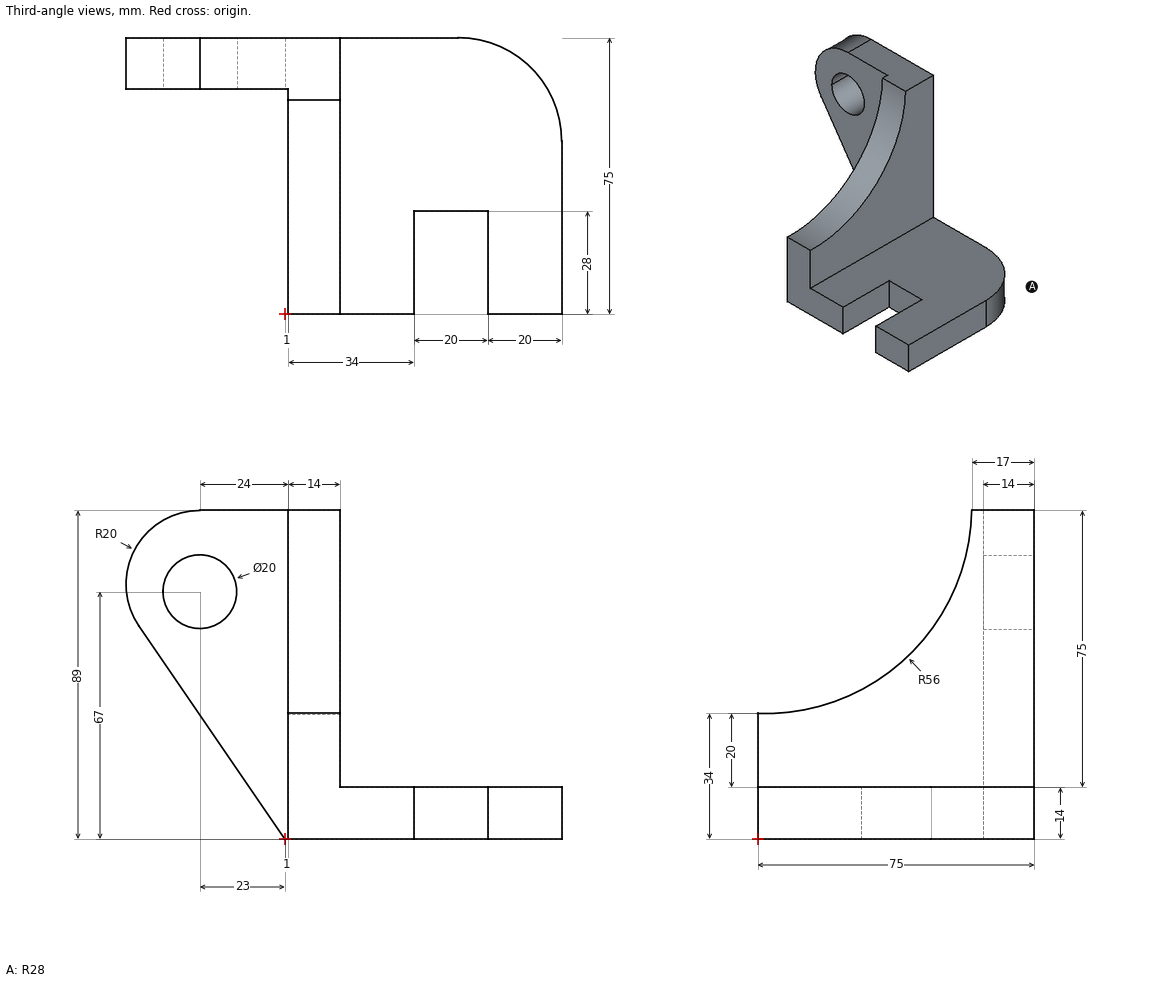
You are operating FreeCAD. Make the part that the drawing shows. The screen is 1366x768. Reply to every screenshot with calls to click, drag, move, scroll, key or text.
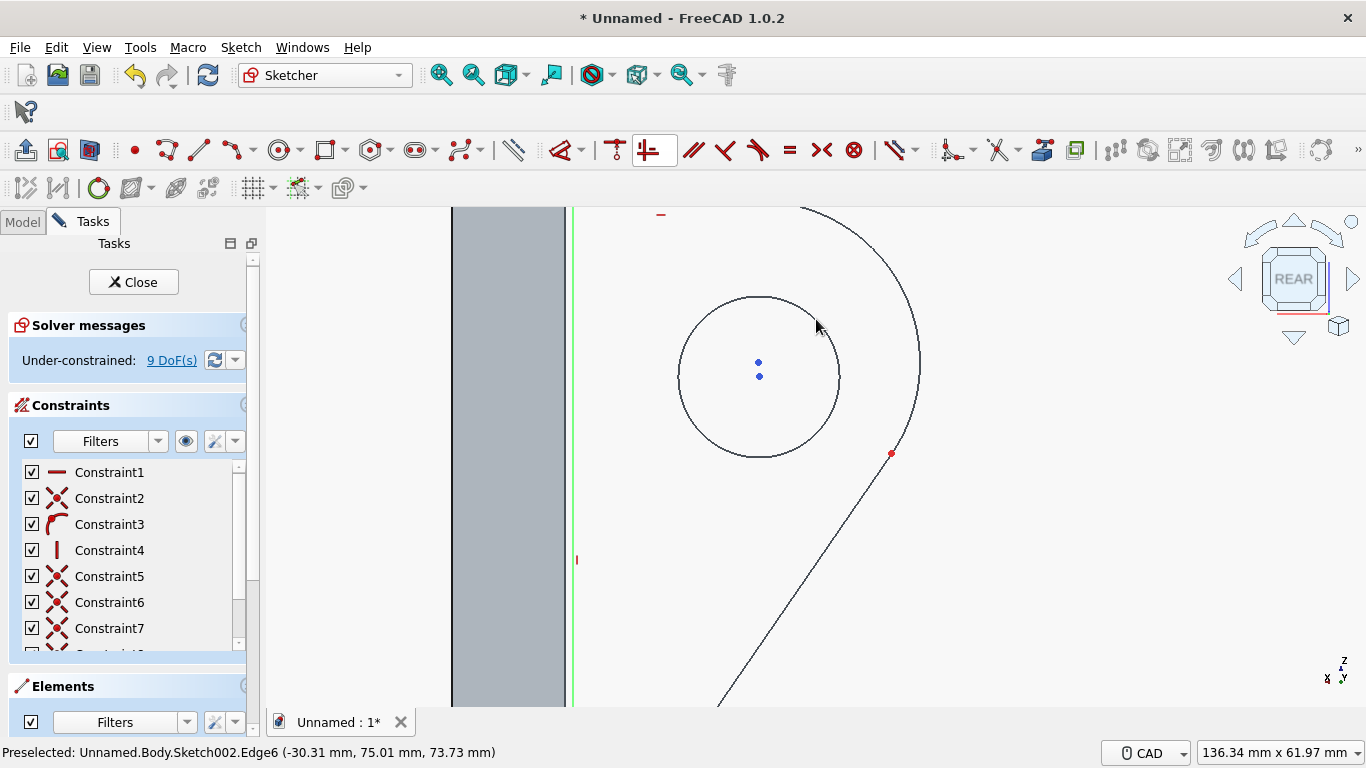
scroll(759, 375, down, 4)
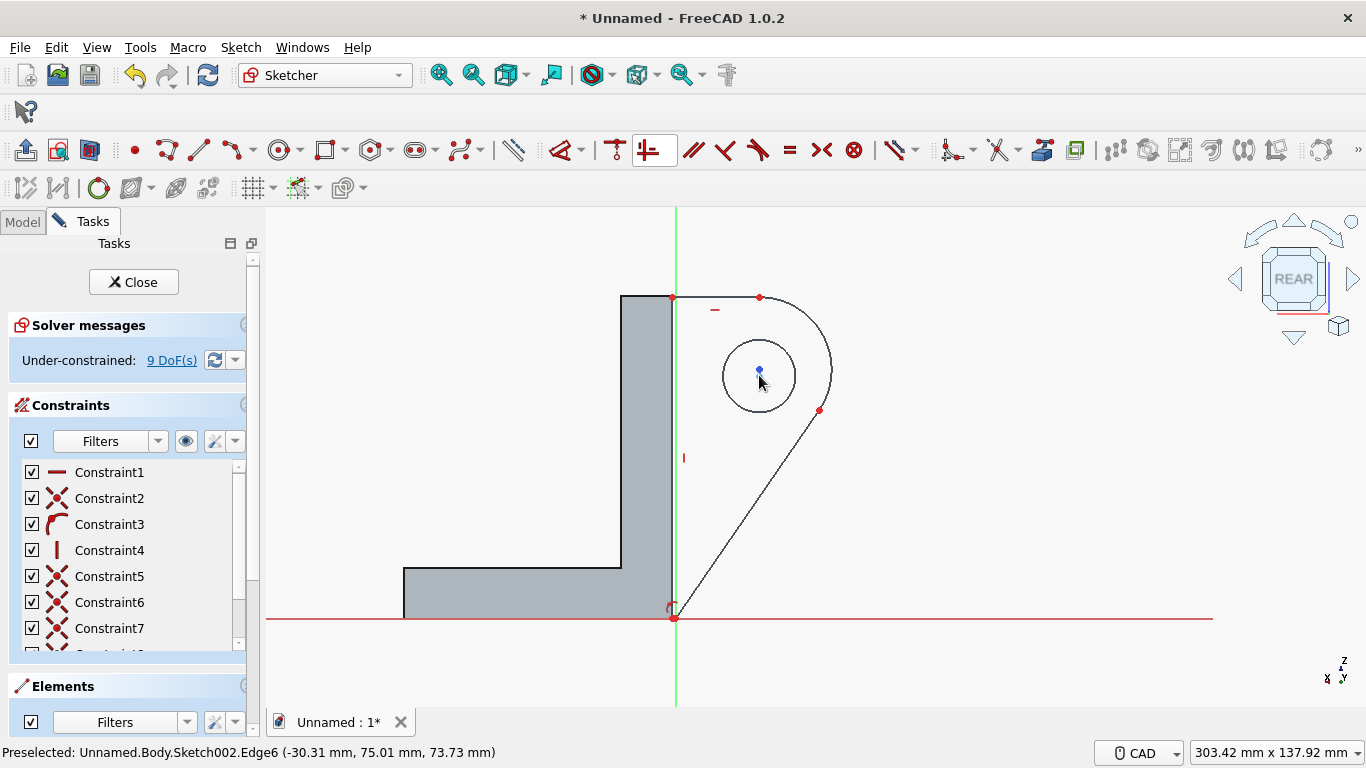
click(733, 297)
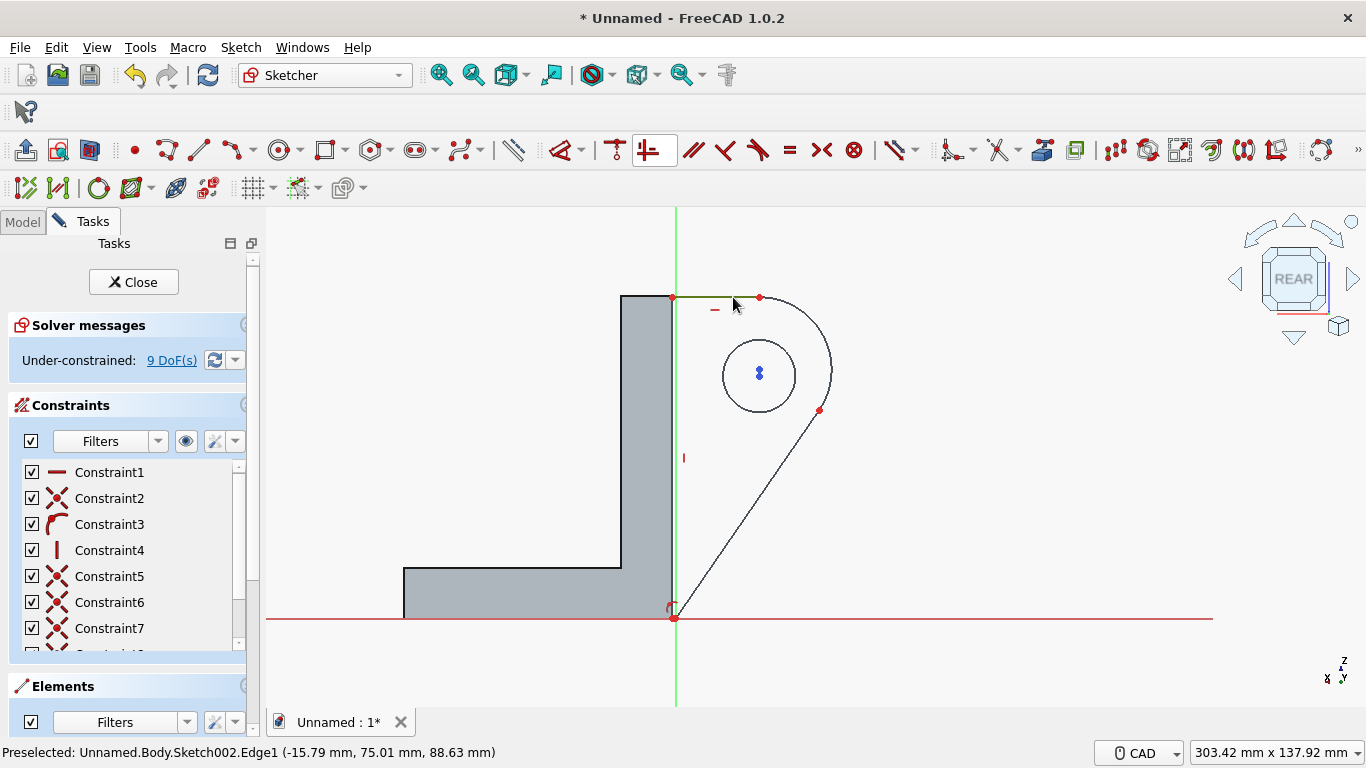
click(831, 366)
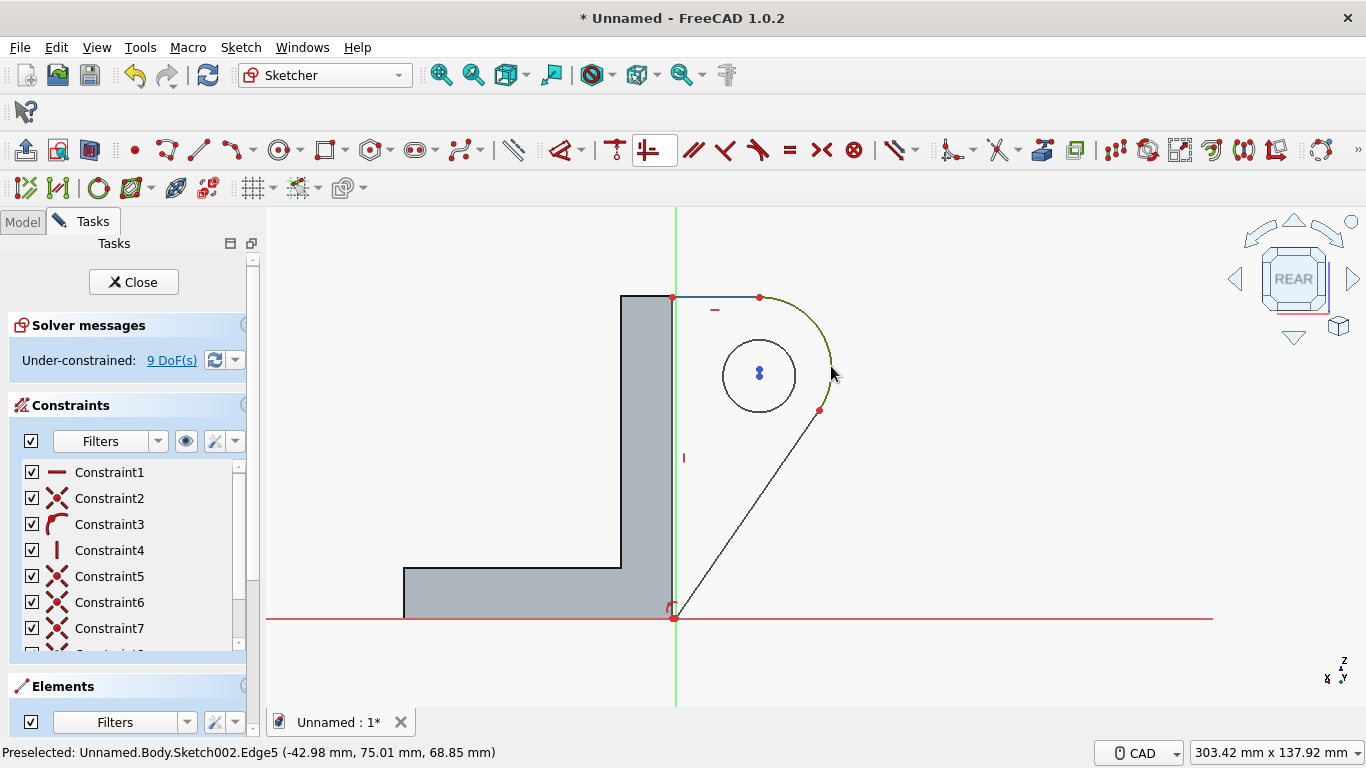
click(758, 150)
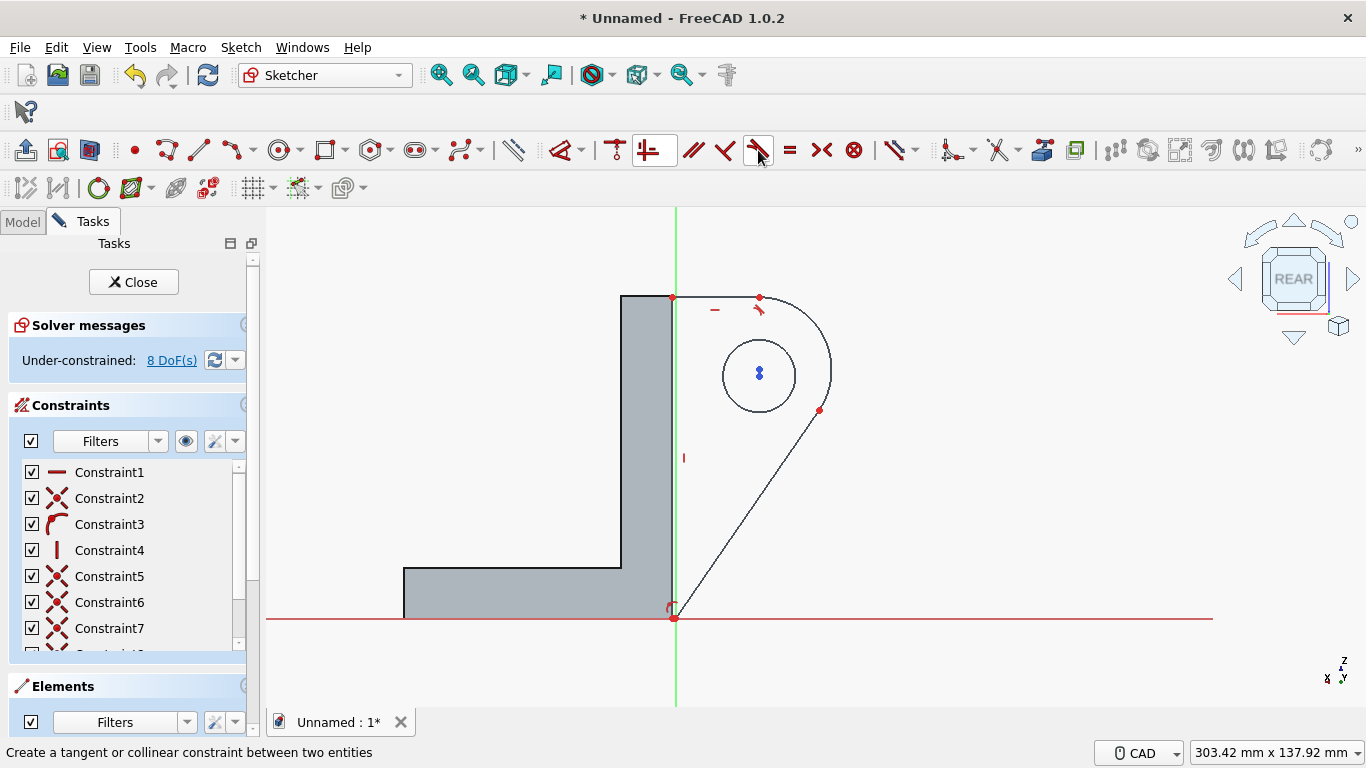
click(719, 556)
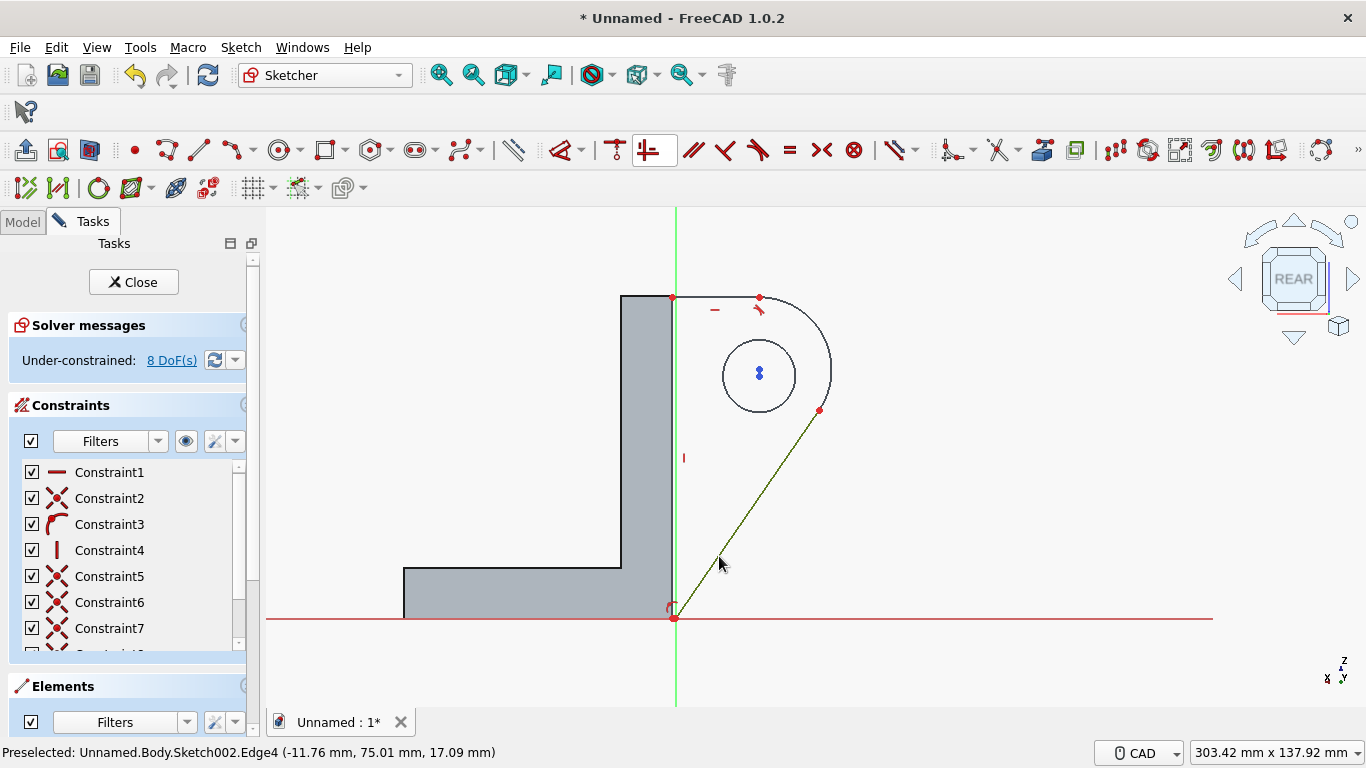
click(831, 366)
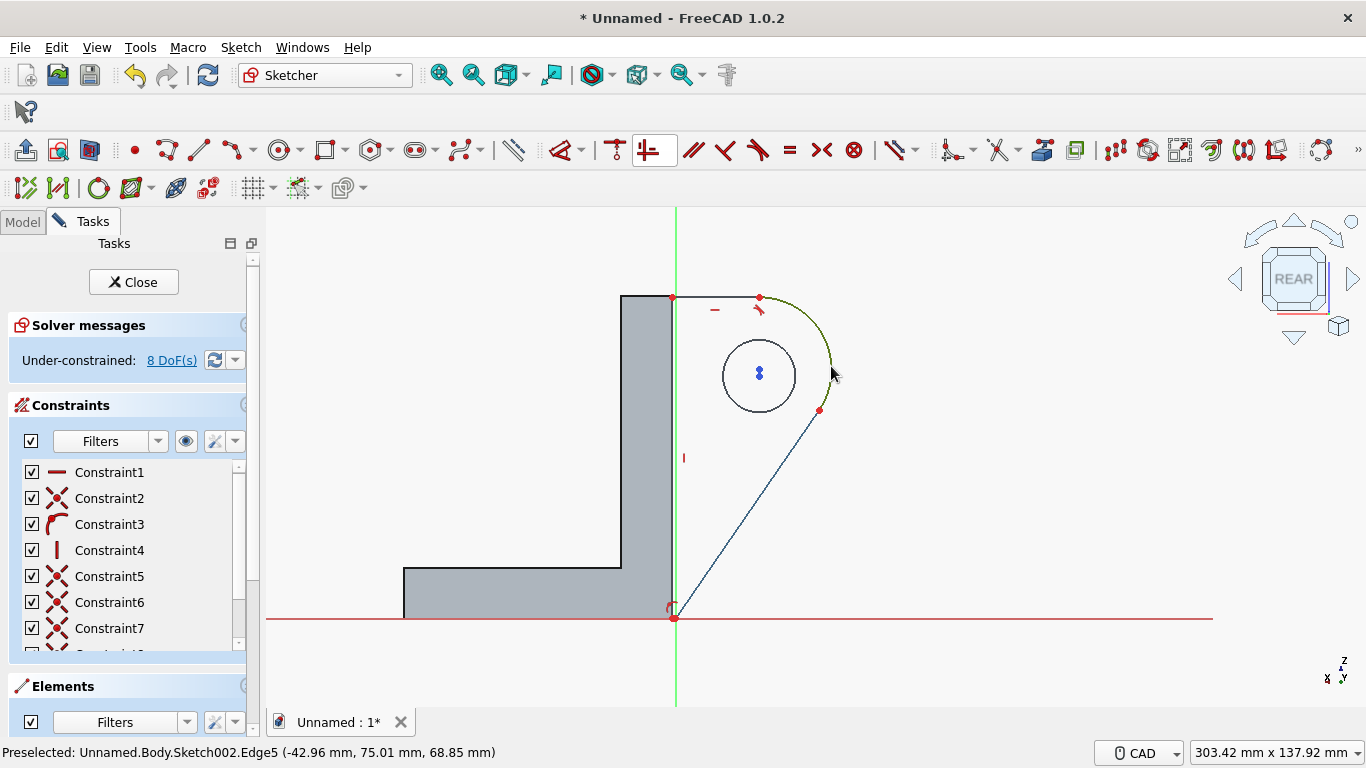
click(758, 150)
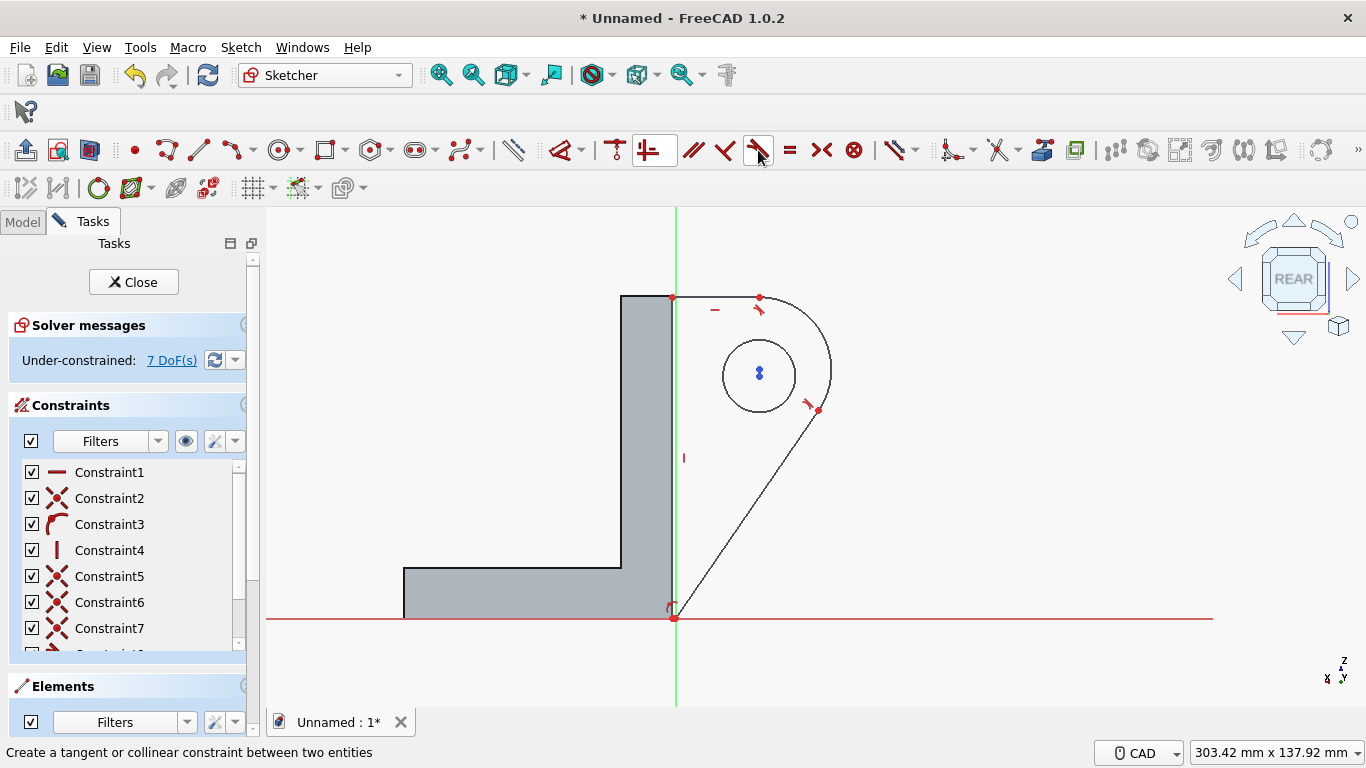
click(560, 150)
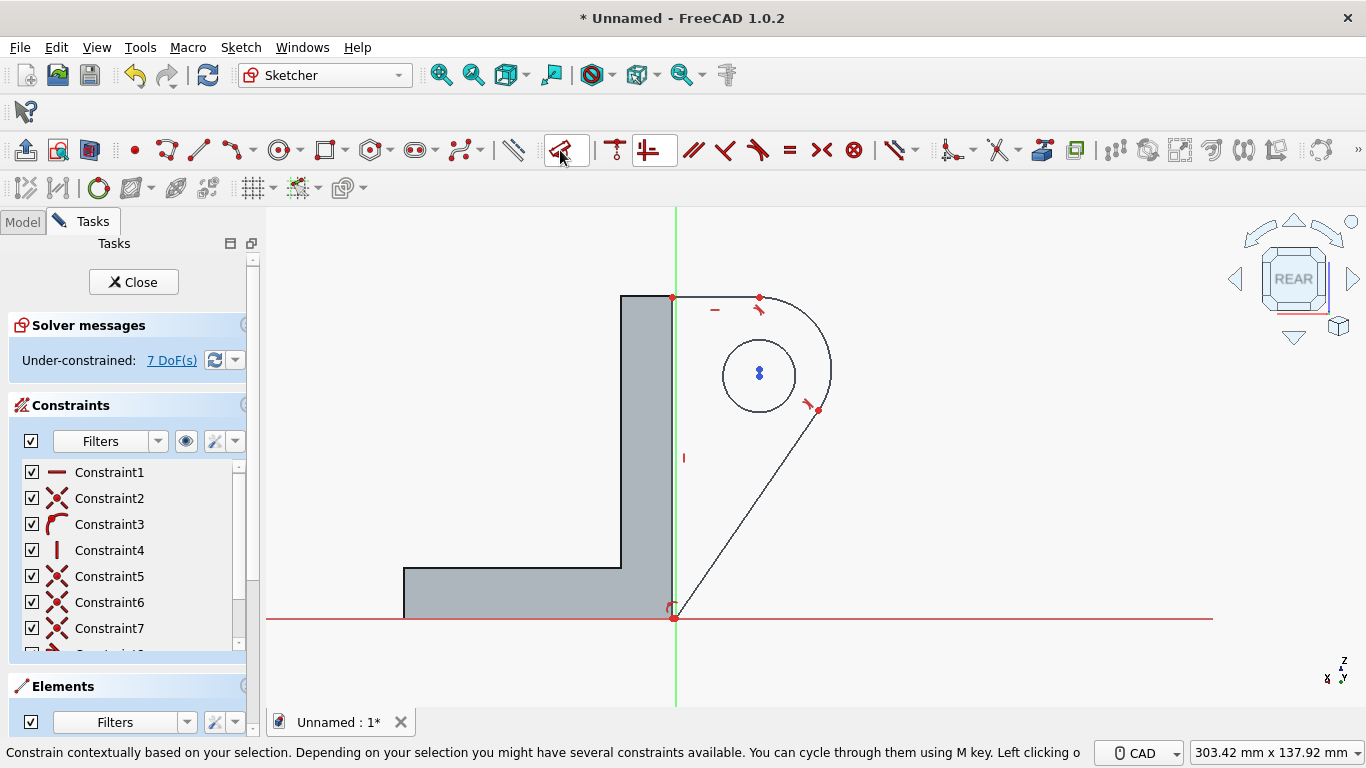
click(831, 366)
click(863, 364)